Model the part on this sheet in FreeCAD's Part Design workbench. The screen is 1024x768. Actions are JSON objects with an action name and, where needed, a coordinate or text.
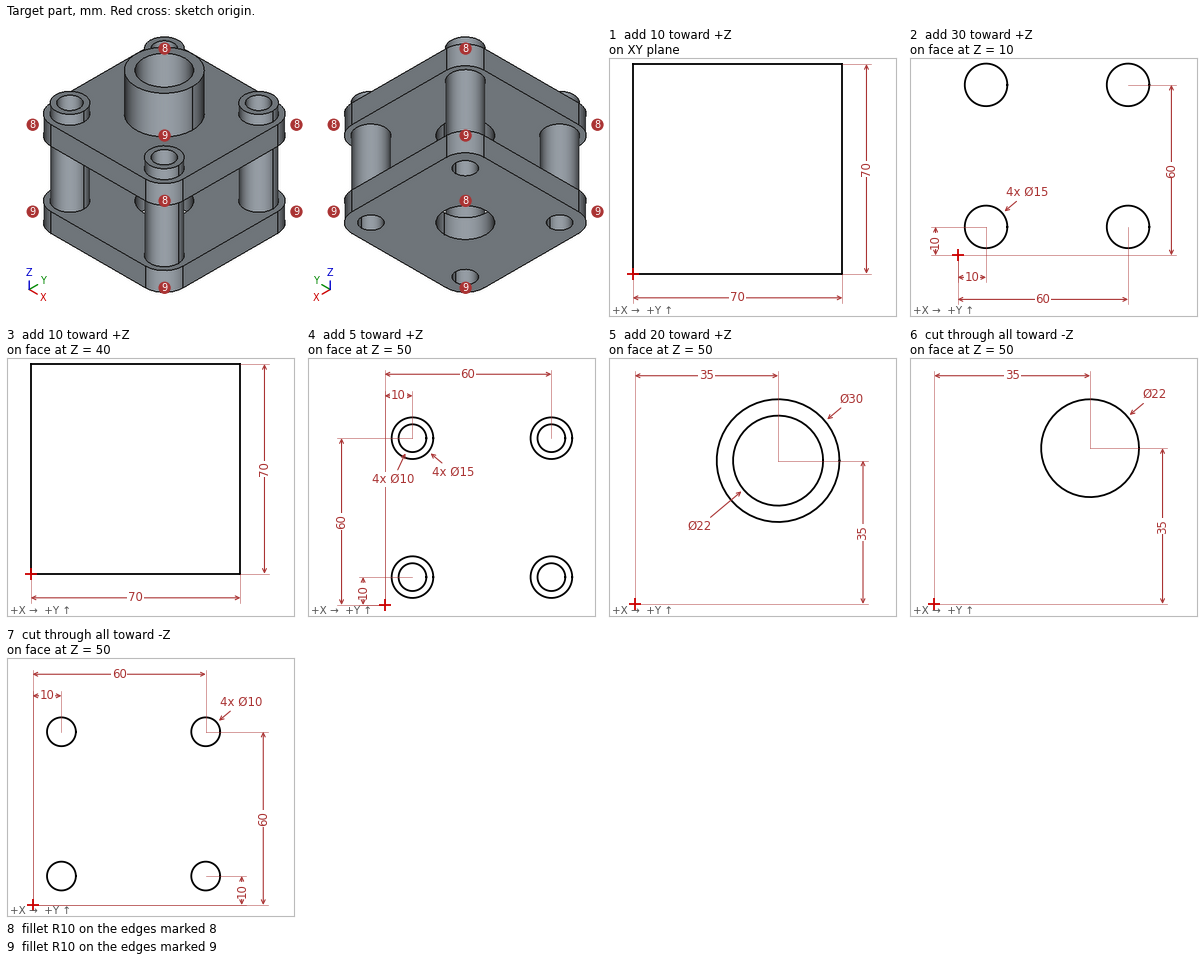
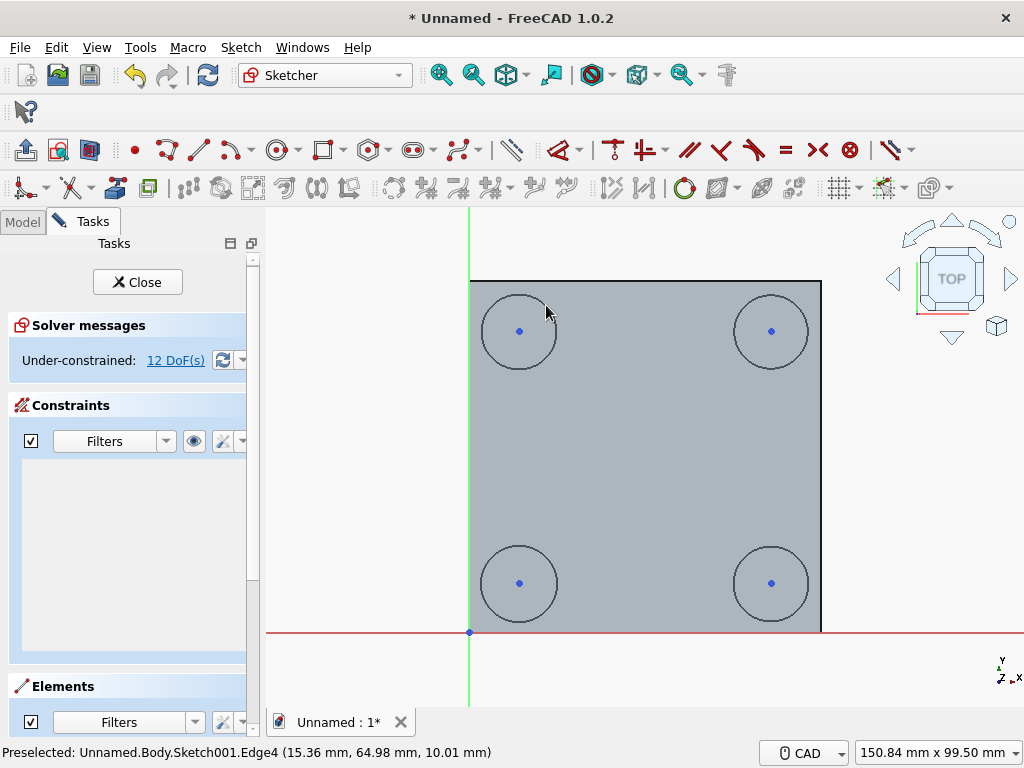
{"action": "left_click", "coordinate": [546, 557]}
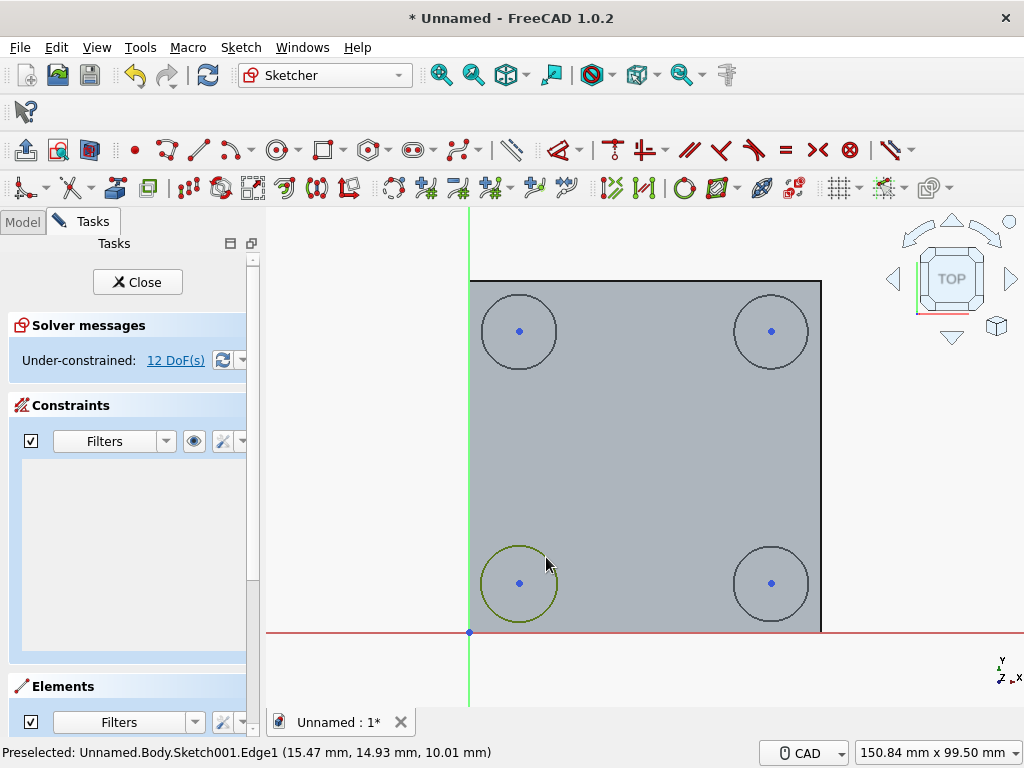
{"action": "left_click", "coordinate": [797, 557]}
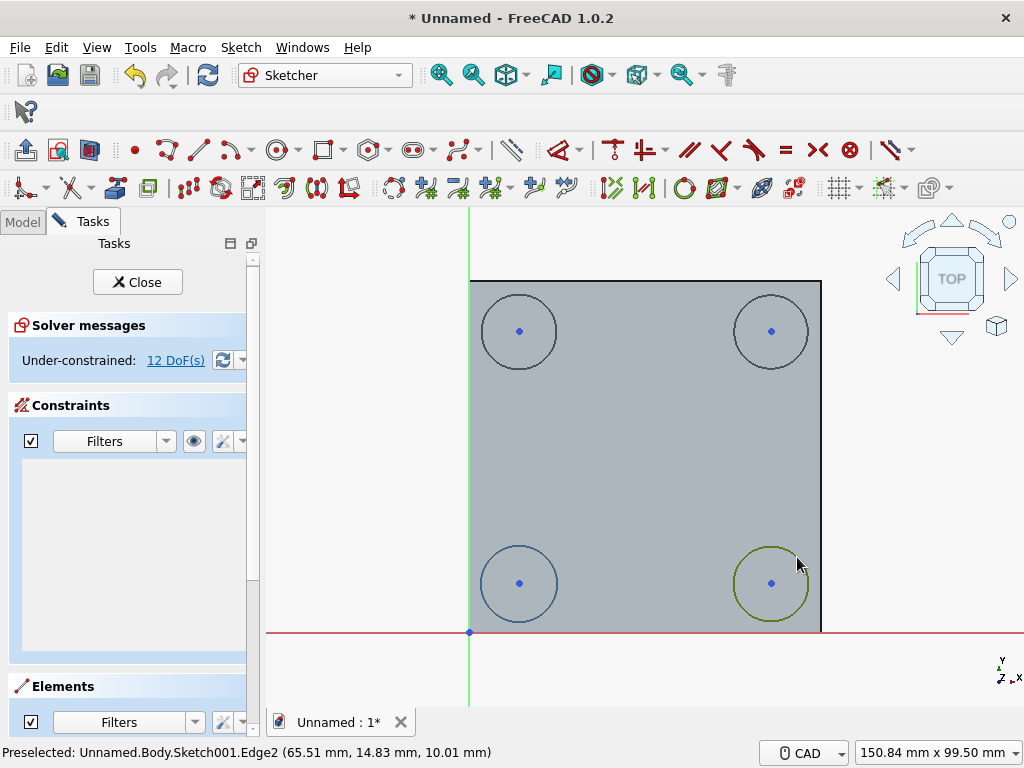
{"action": "left_click", "coordinate": [797, 306]}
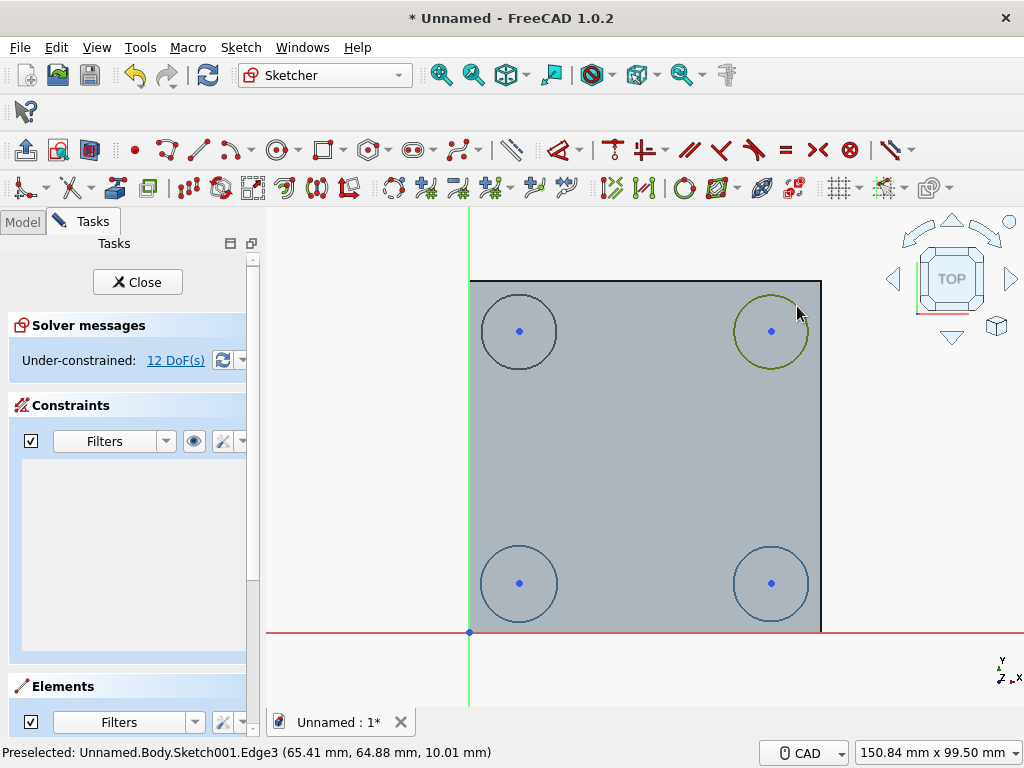
{"action": "left_click", "coordinate": [545, 305]}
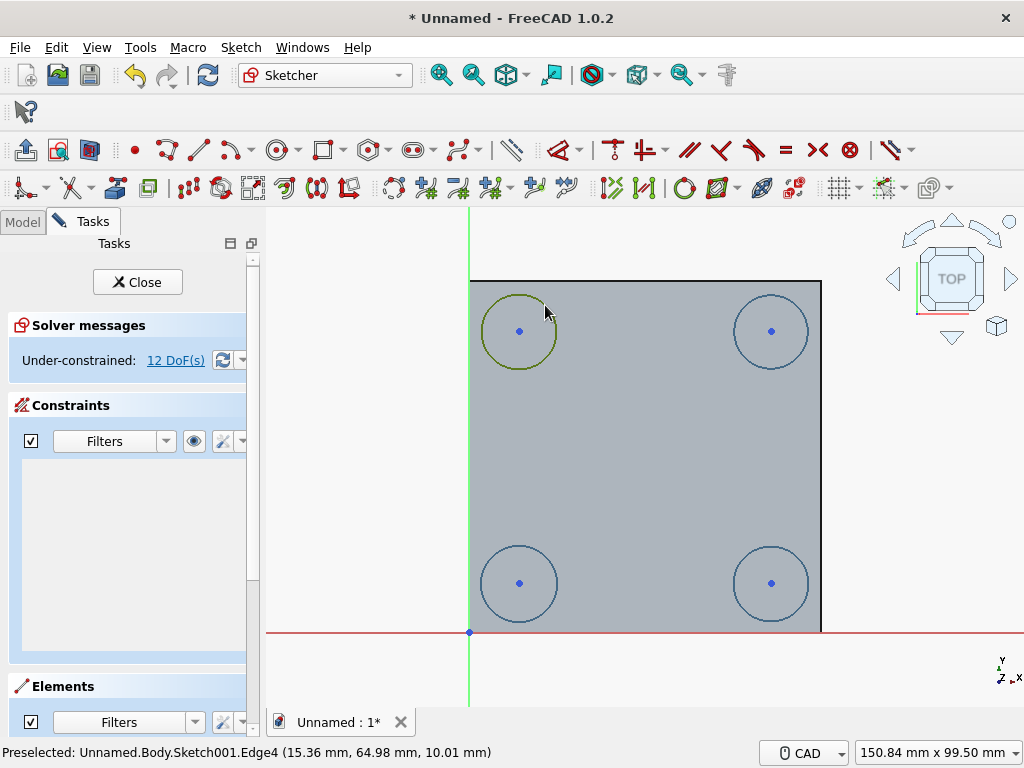
{"action": "key", "text": "e"}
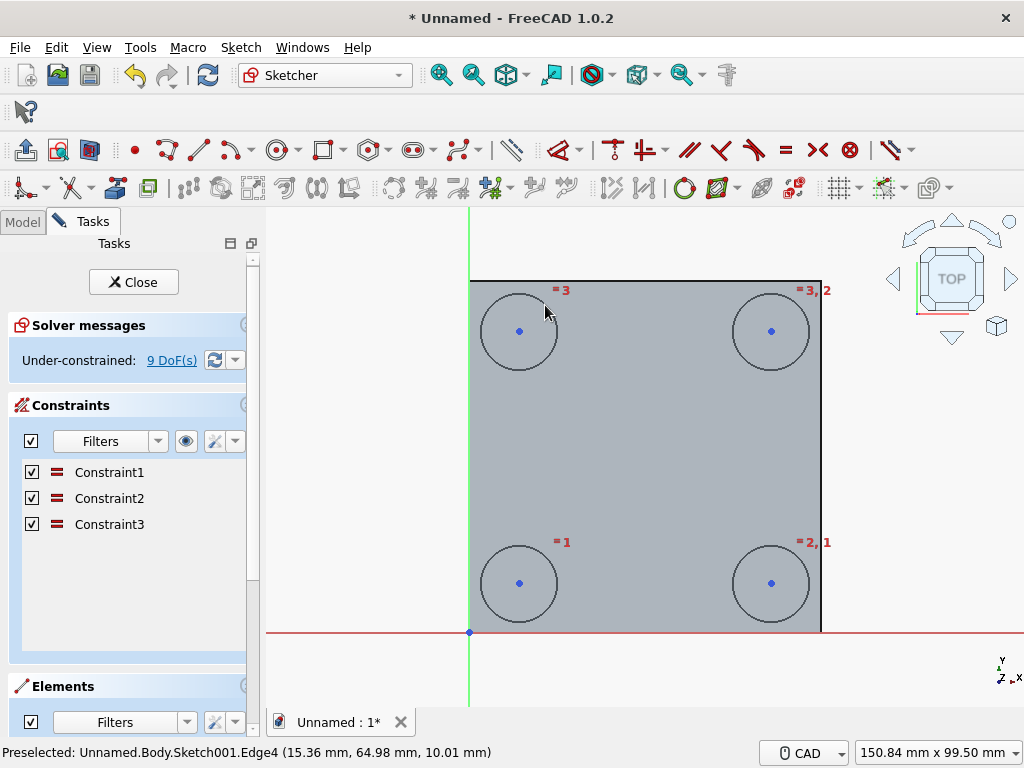
{"action": "left_click", "coordinate": [519, 584]}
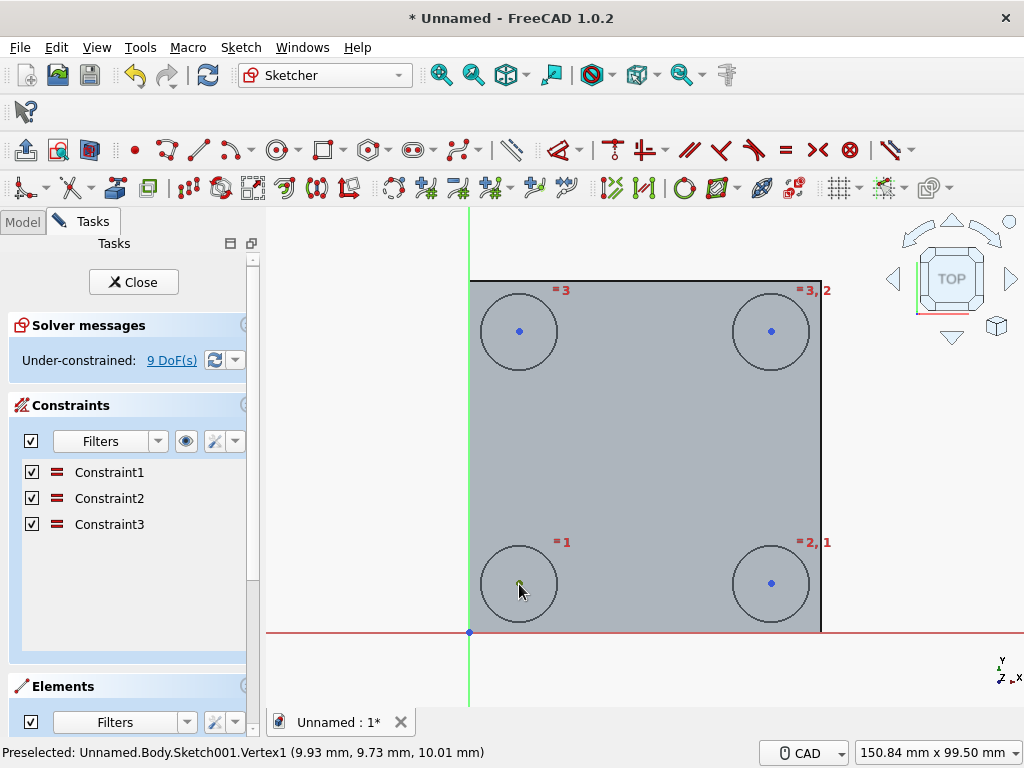
{"action": "left_click", "coordinate": [771, 584]}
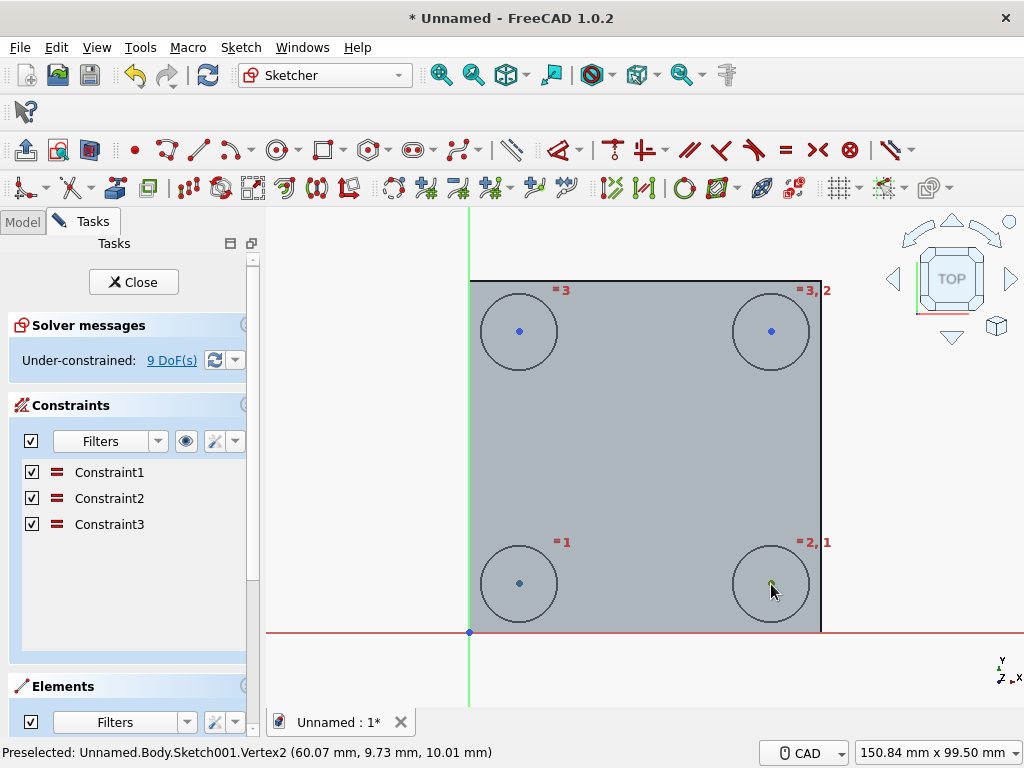
{"action": "key", "text": "h"}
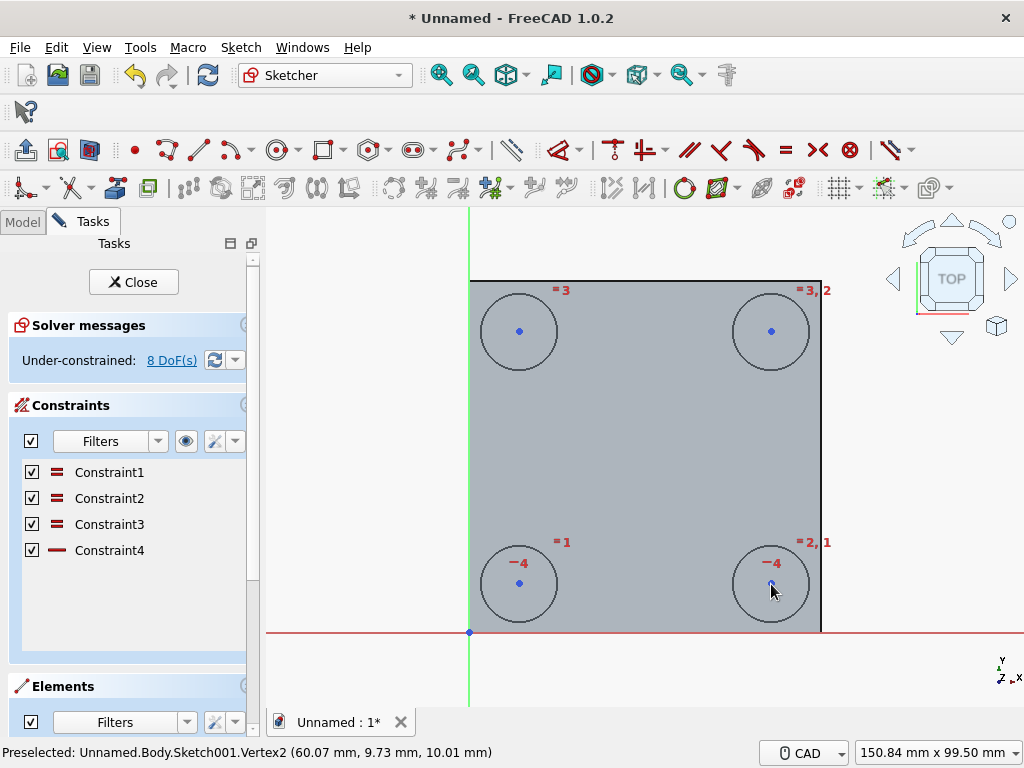
{"action": "left_click", "coordinate": [771, 584]}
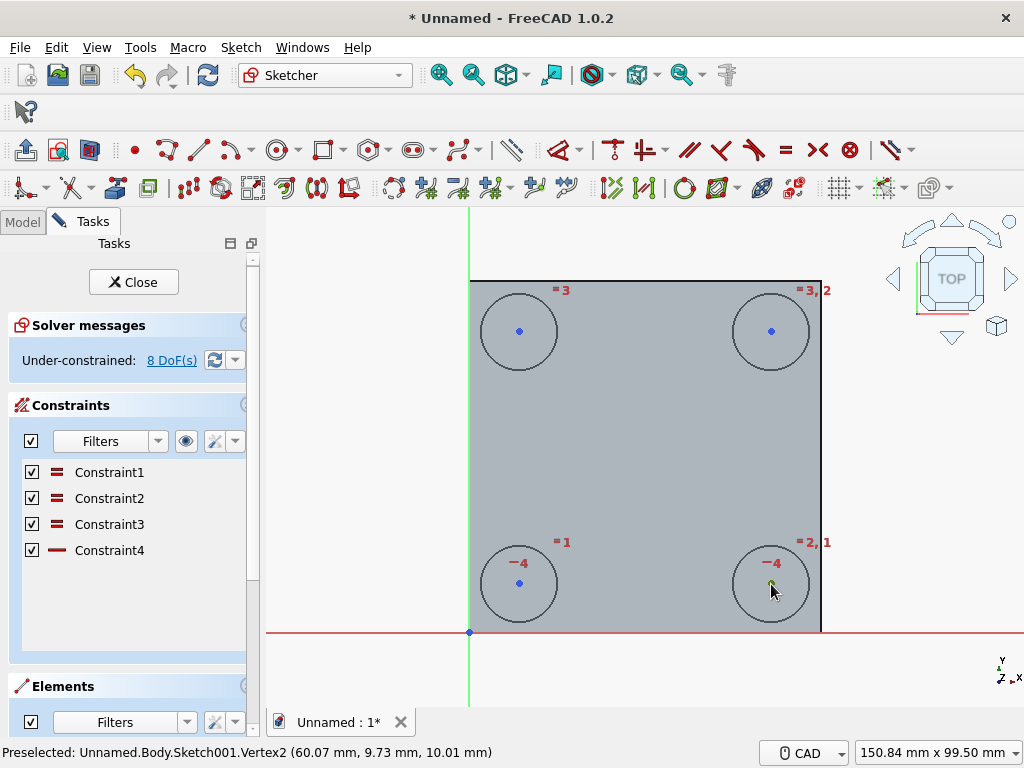
{"action": "left_click", "coordinate": [771, 332]}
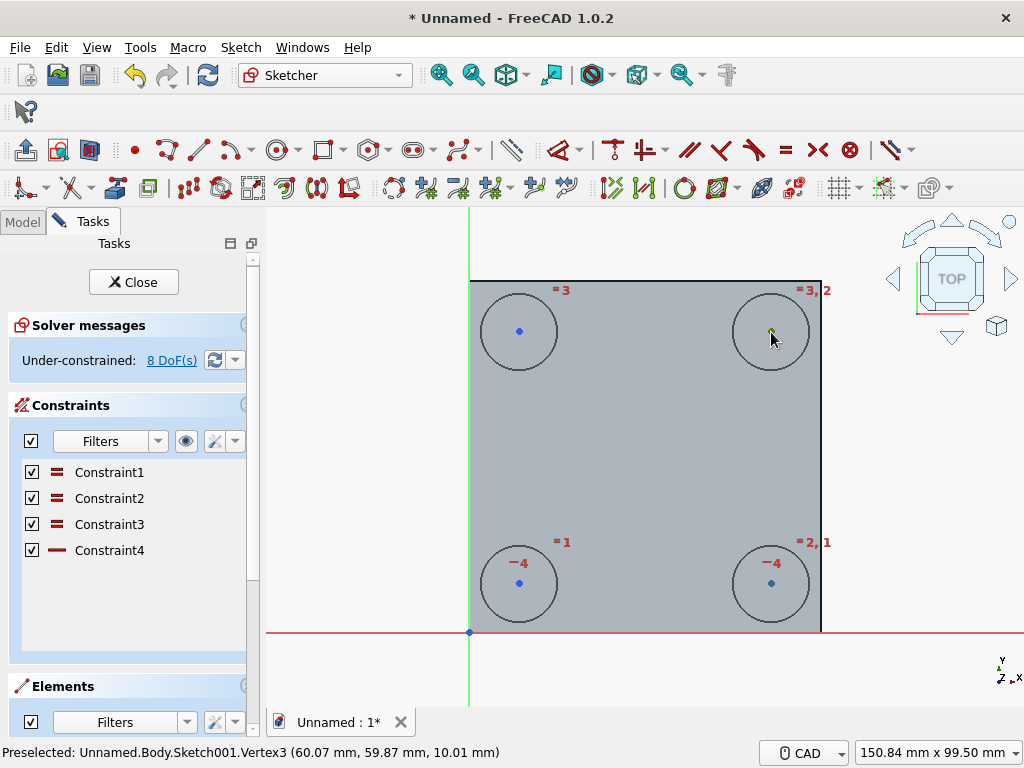
{"action": "key", "text": "v"}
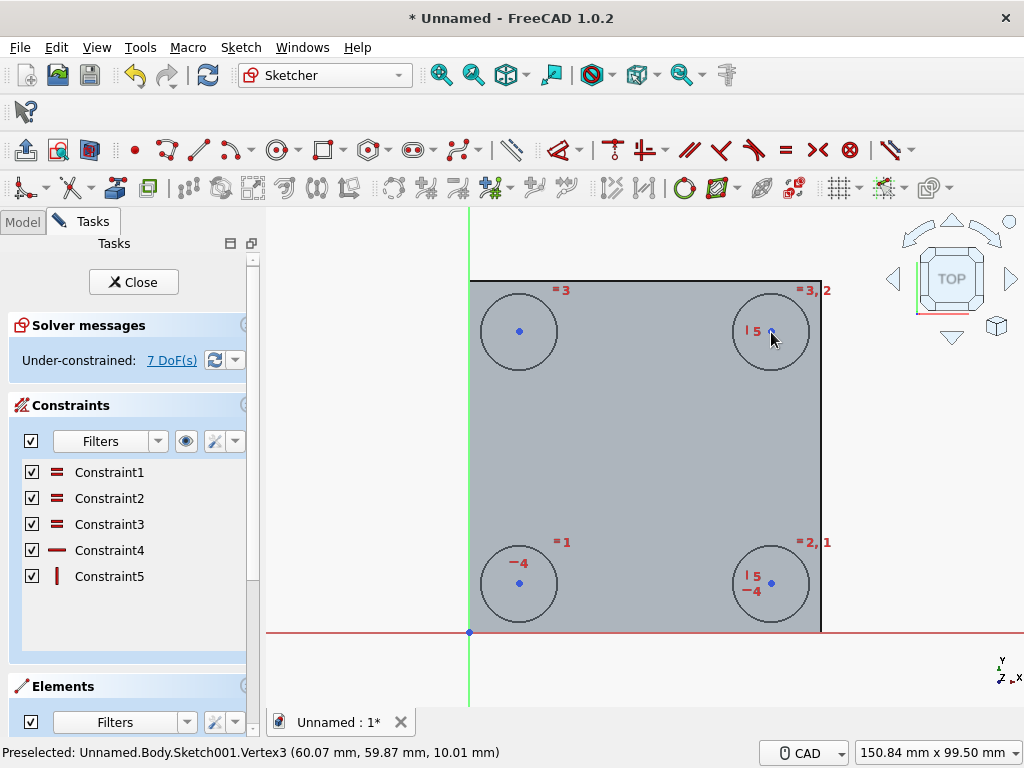
{"action": "left_click", "coordinate": [519, 584]}